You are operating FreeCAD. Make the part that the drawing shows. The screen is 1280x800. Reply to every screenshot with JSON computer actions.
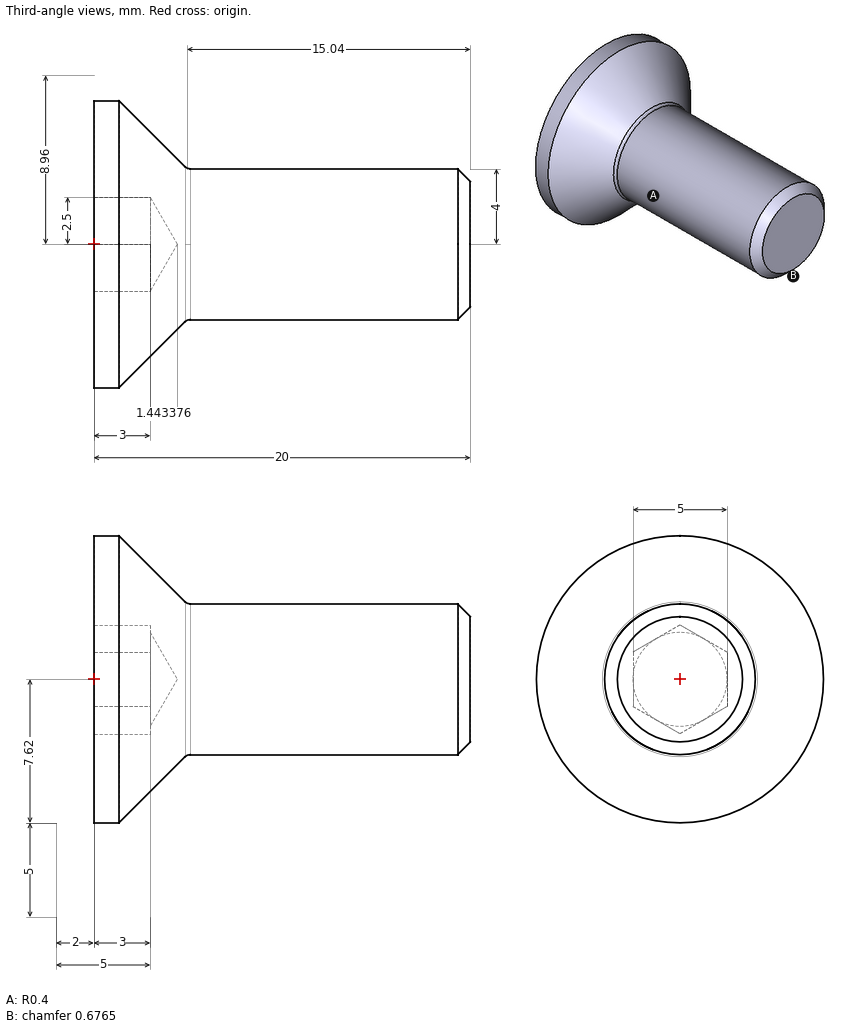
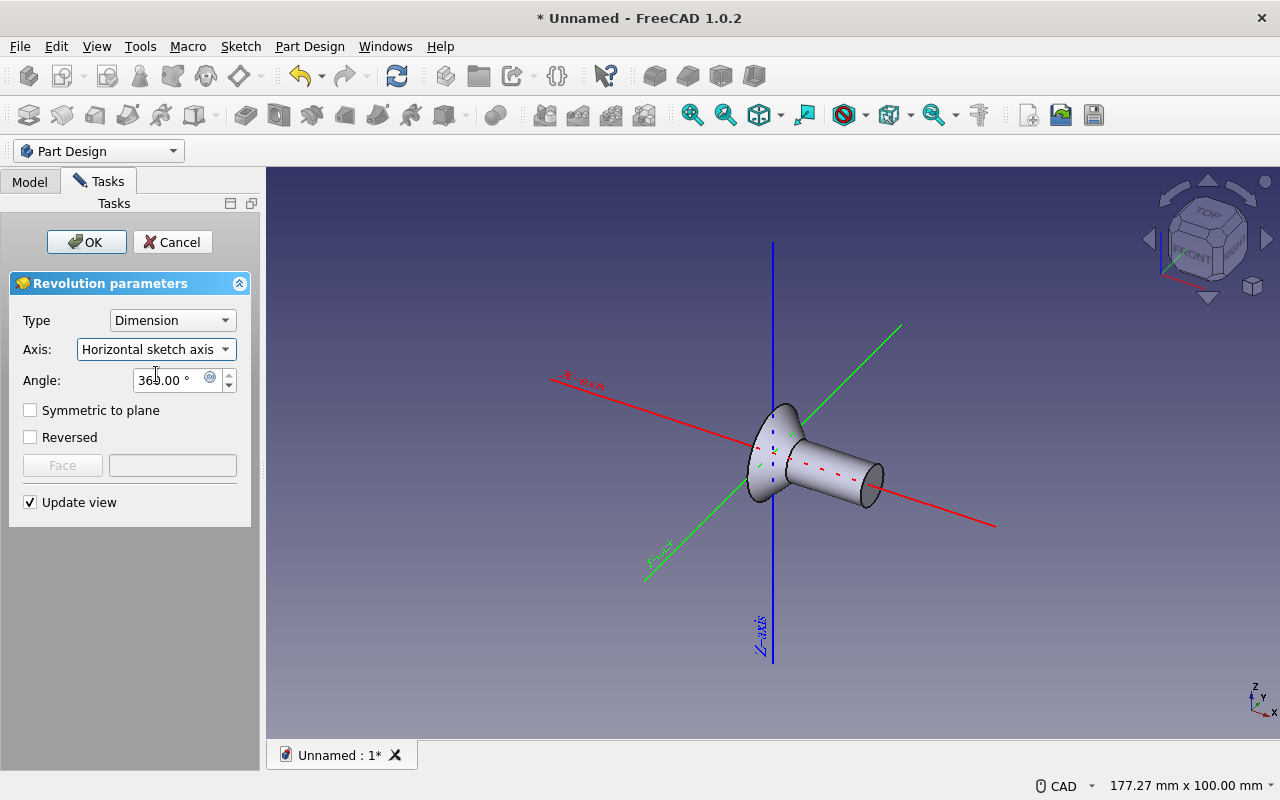
{"action": "left_click", "coordinate": [87, 242]}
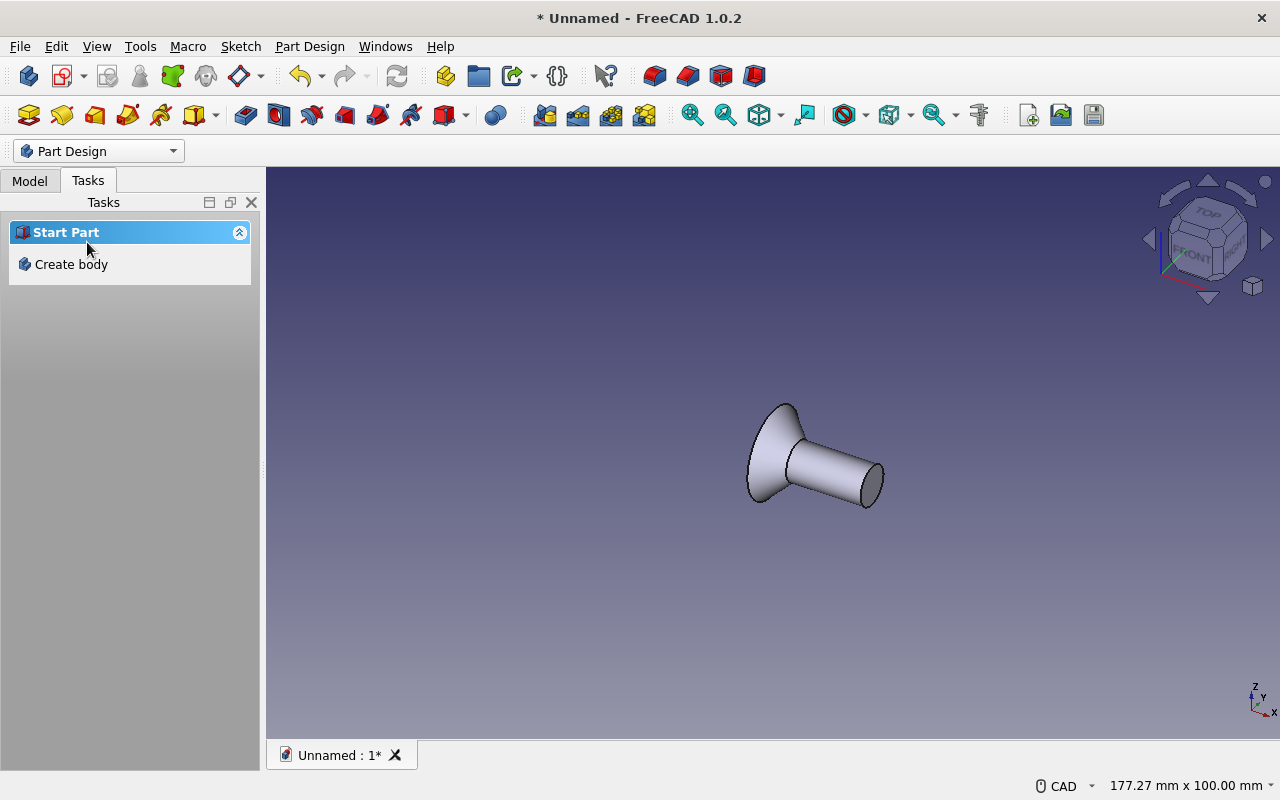
{"action": "left_click", "coordinate": [693, 116]}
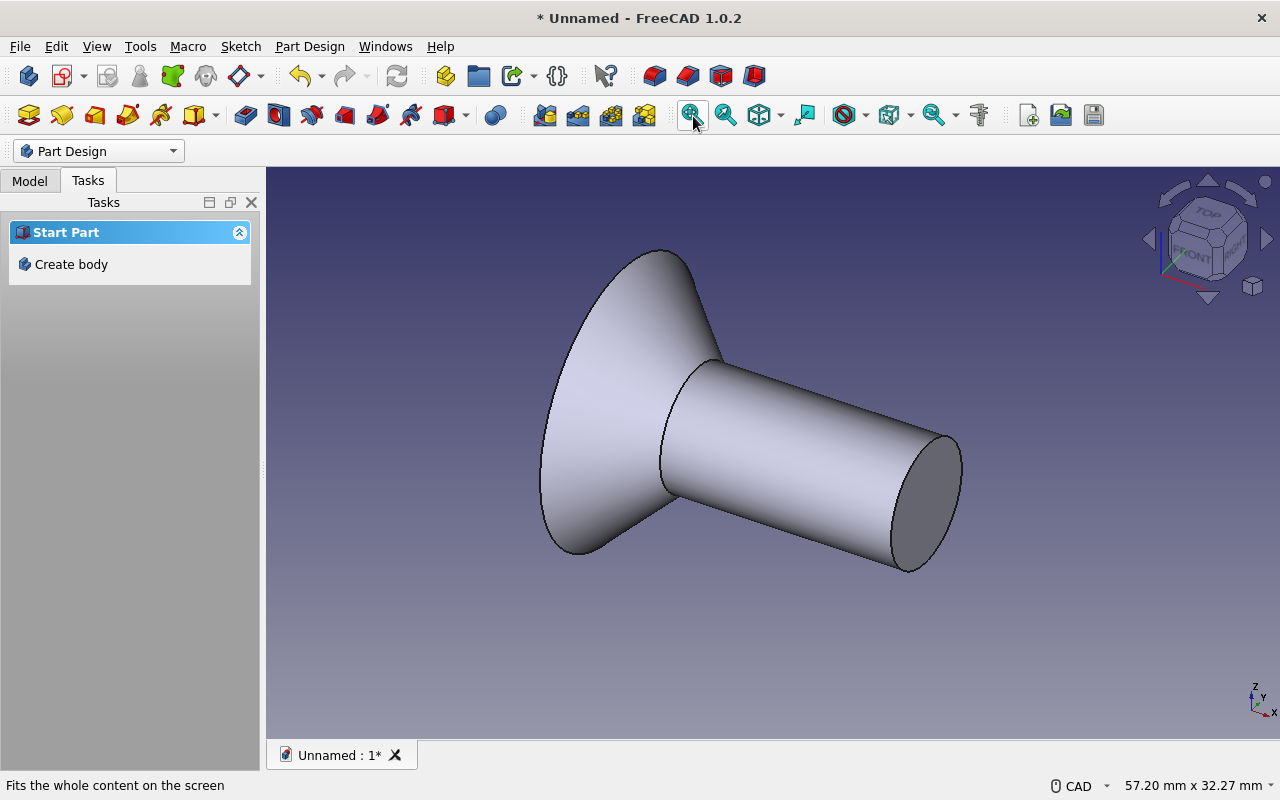
{"action": "left_click", "coordinate": [62, 76]}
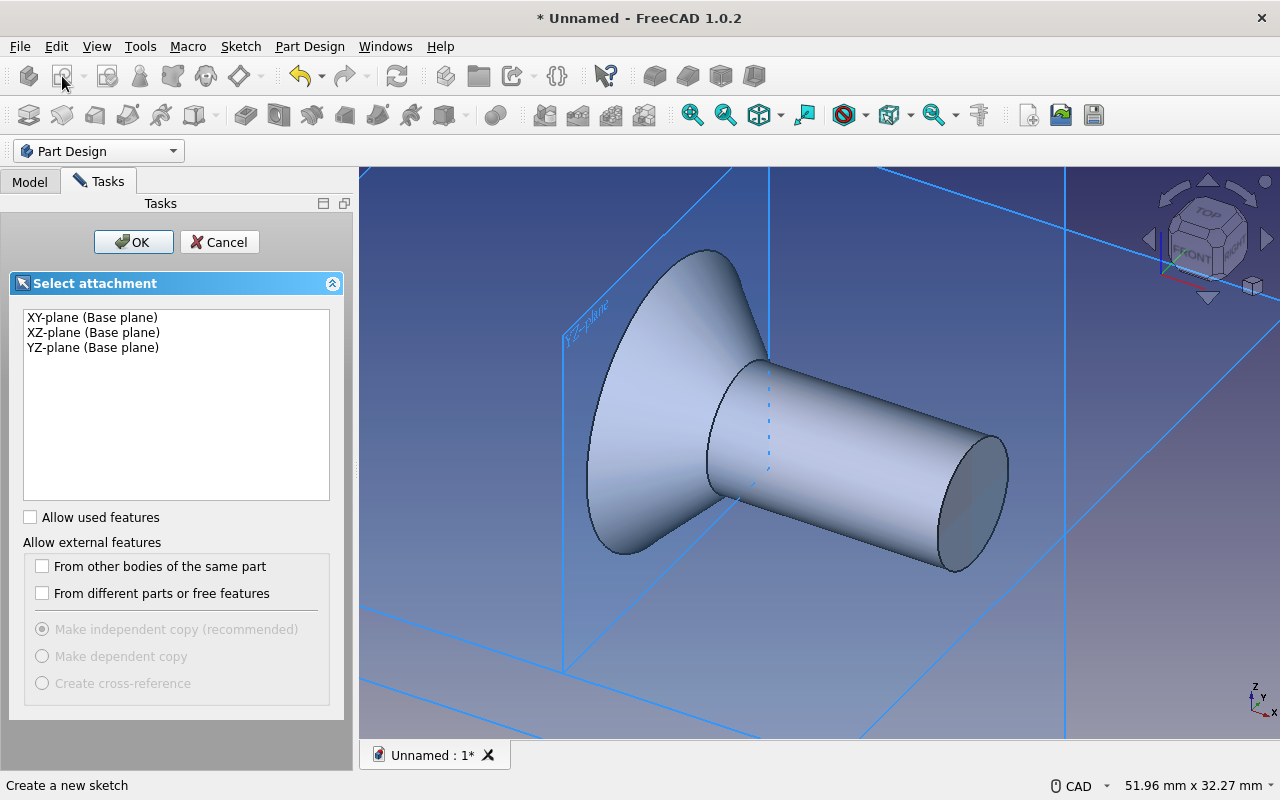
{"action": "left_click", "coordinate": [84, 348]}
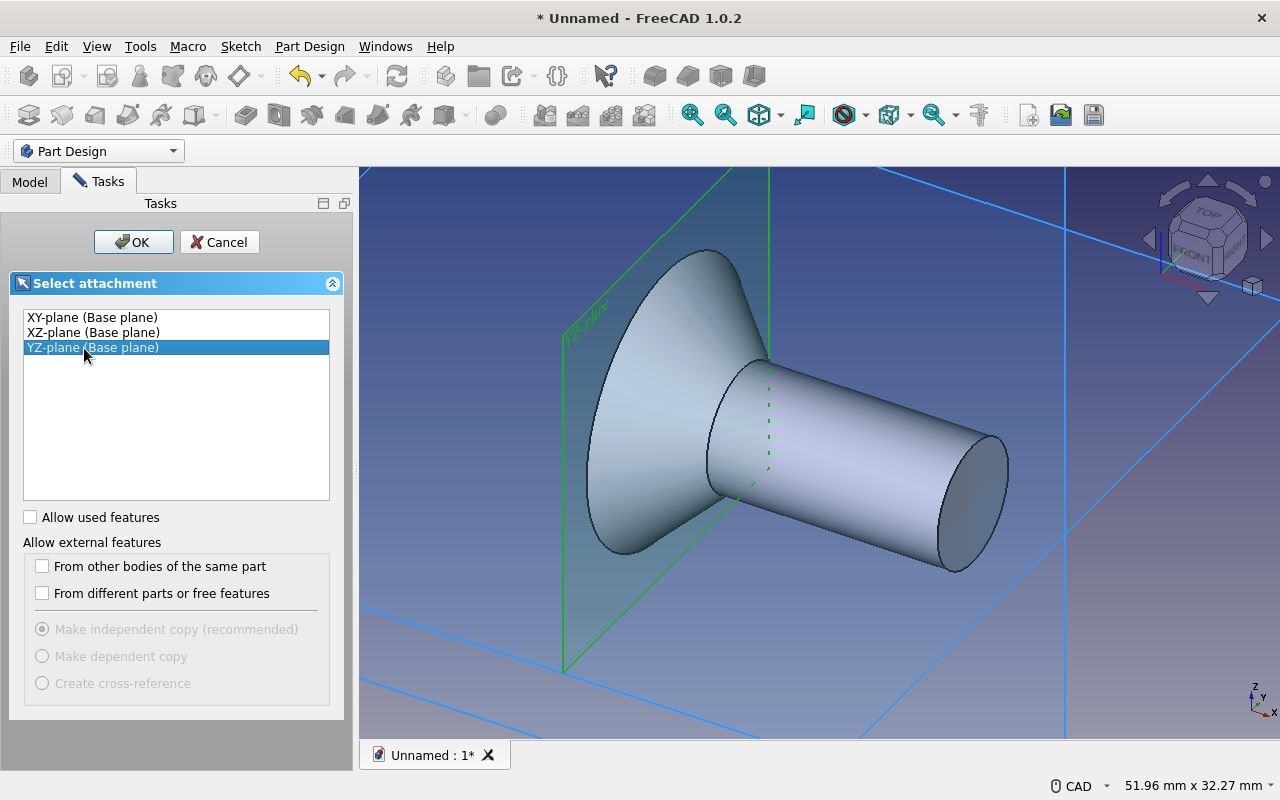
{"action": "left_click", "coordinate": [134, 242]}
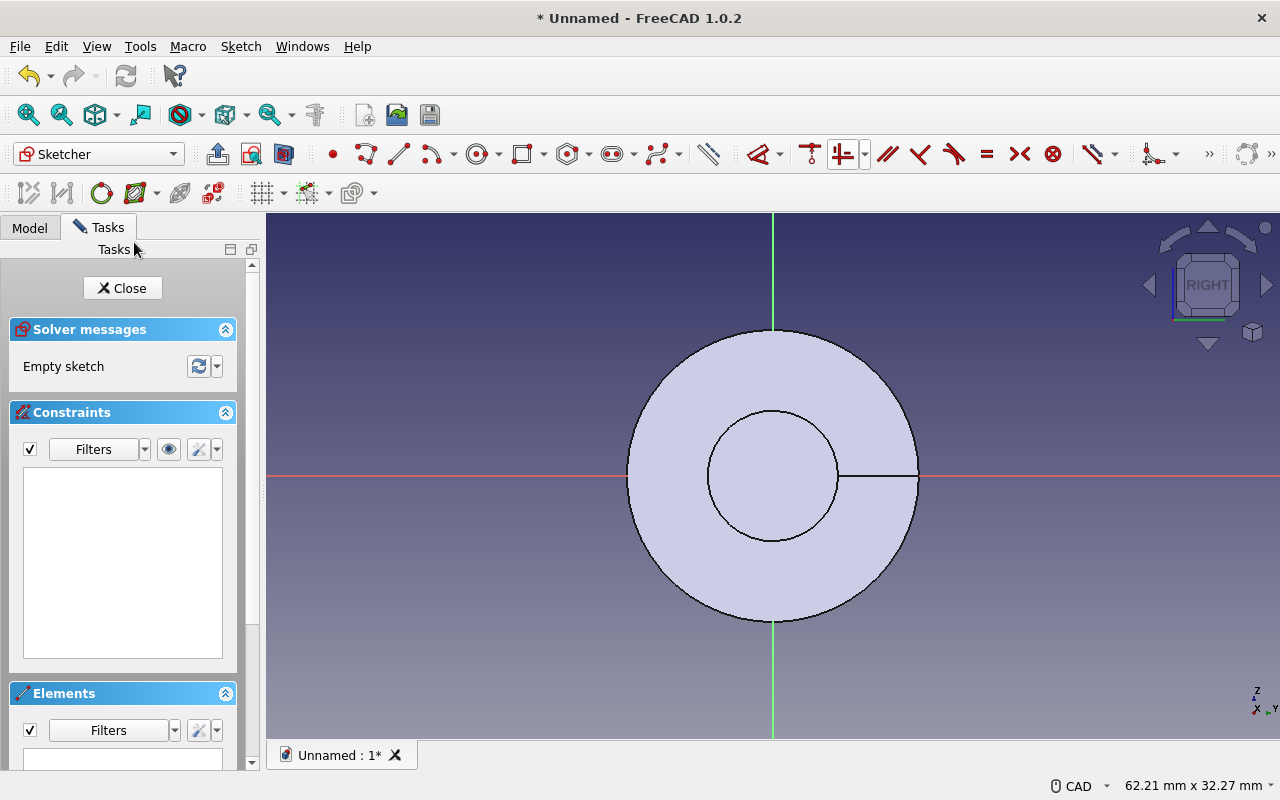
{"action": "left_click", "coordinate": [284, 154]}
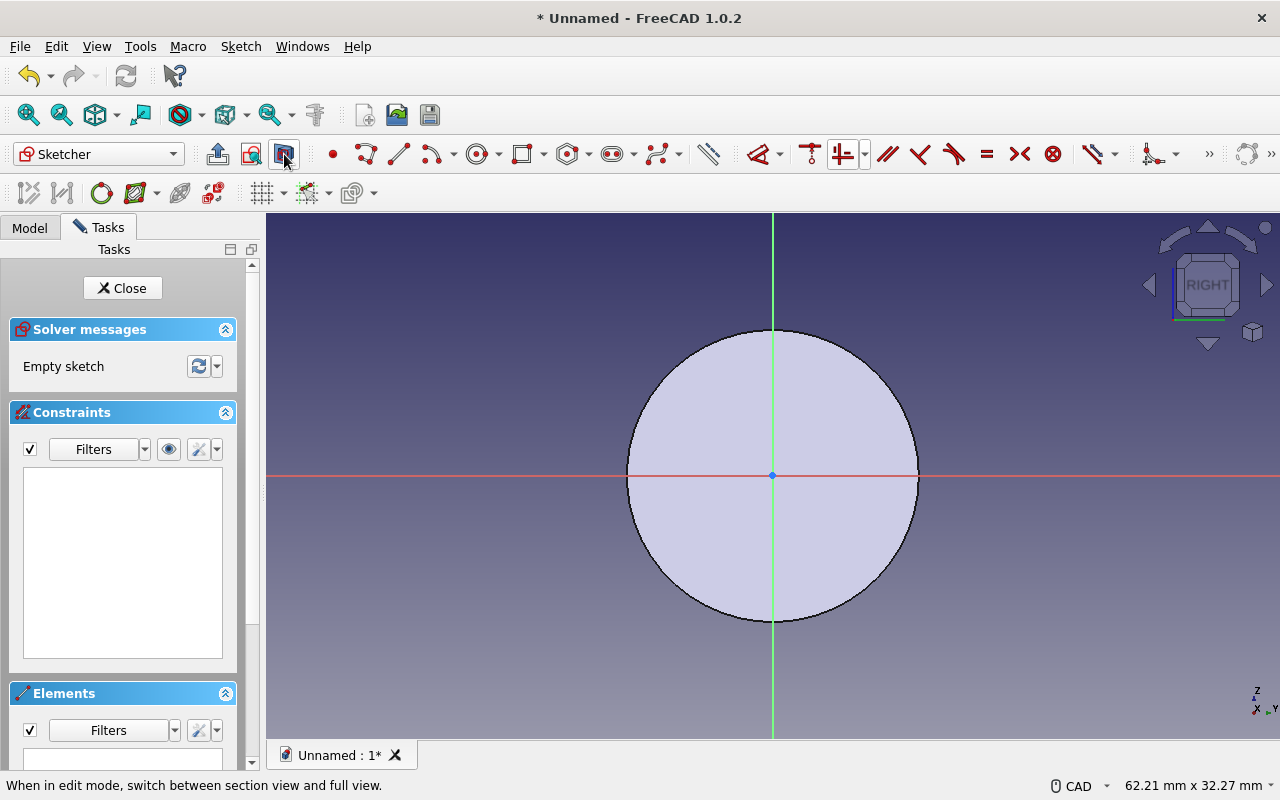
{"action": "scroll", "coordinate": [802, 476], "scroll_direction": "up", "scroll_amount": 6}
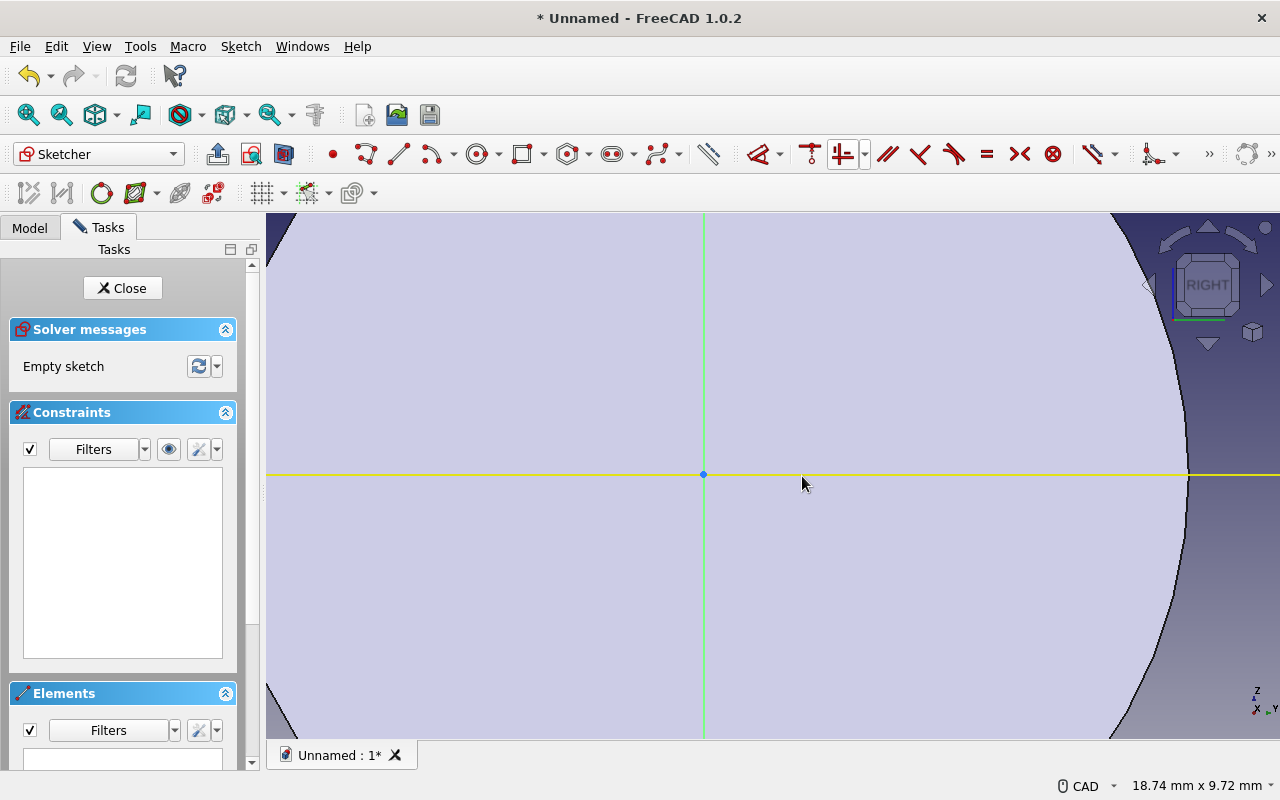
{"action": "left_click", "coordinate": [566, 154]}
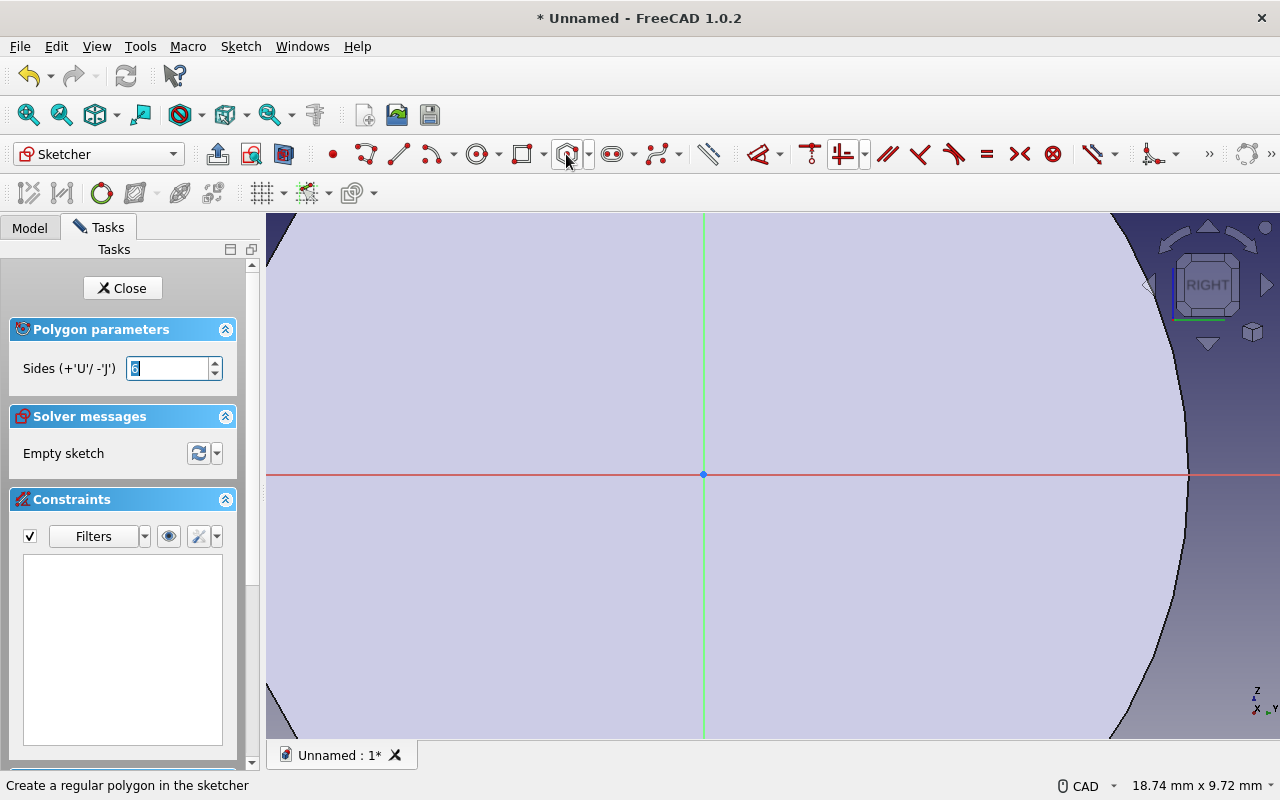
{"action": "left_click", "coordinate": [704, 475]}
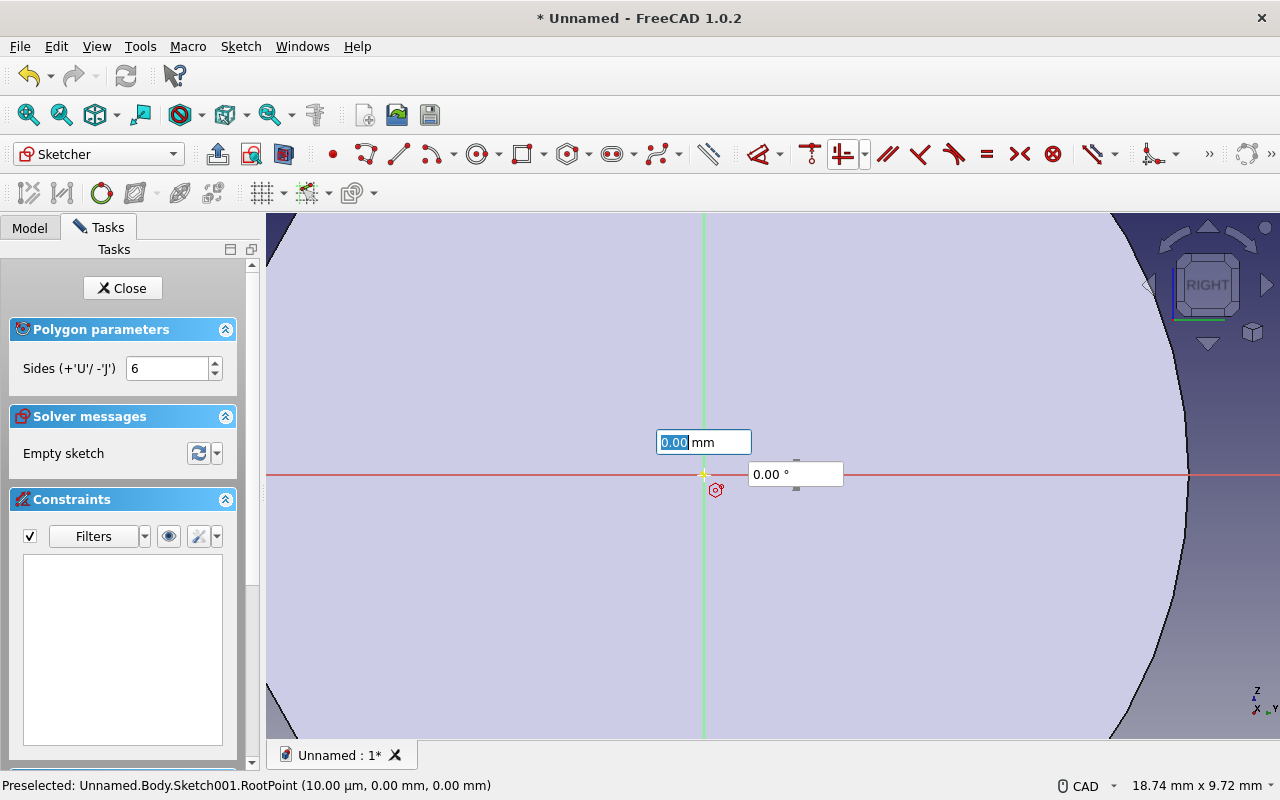
{"action": "left_click", "coordinate": [704, 631]}
{"action": "key", "text": "Escape"}